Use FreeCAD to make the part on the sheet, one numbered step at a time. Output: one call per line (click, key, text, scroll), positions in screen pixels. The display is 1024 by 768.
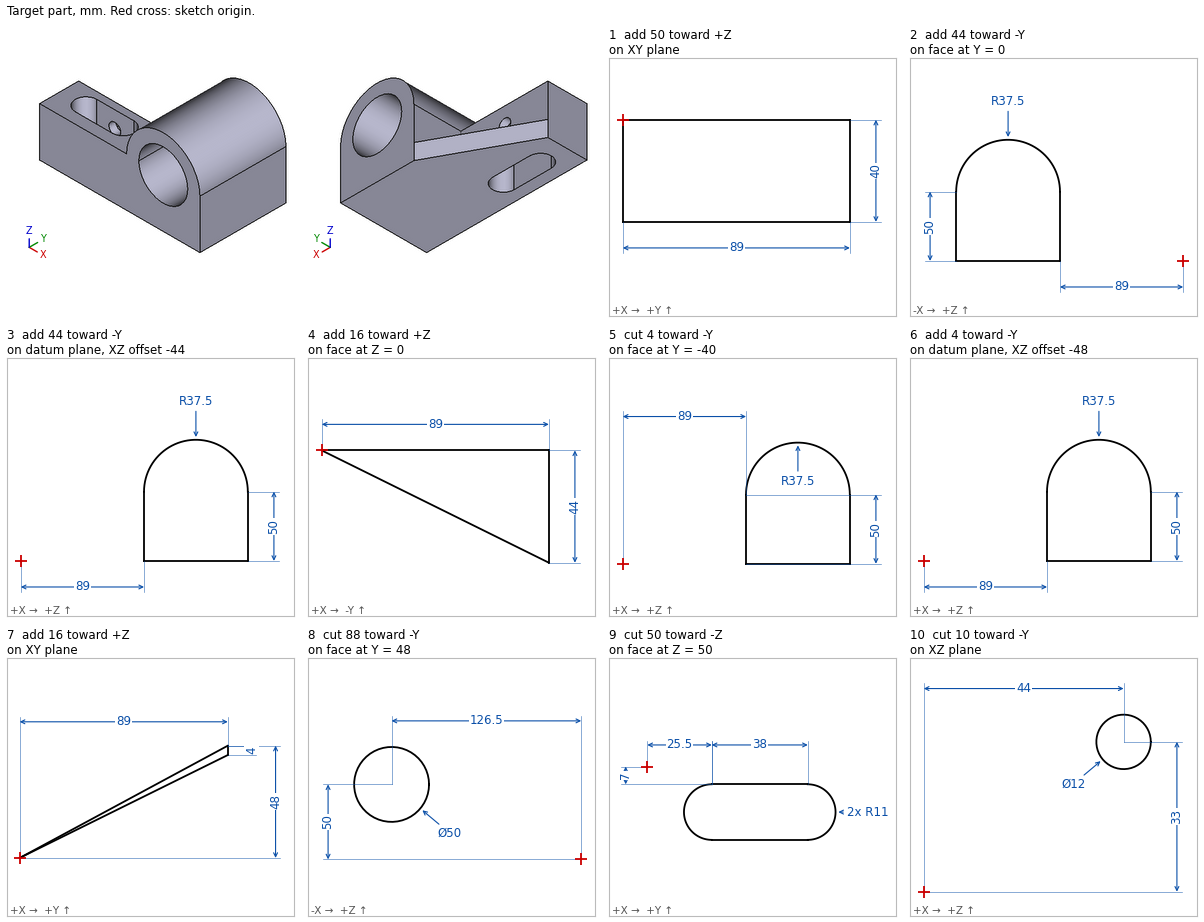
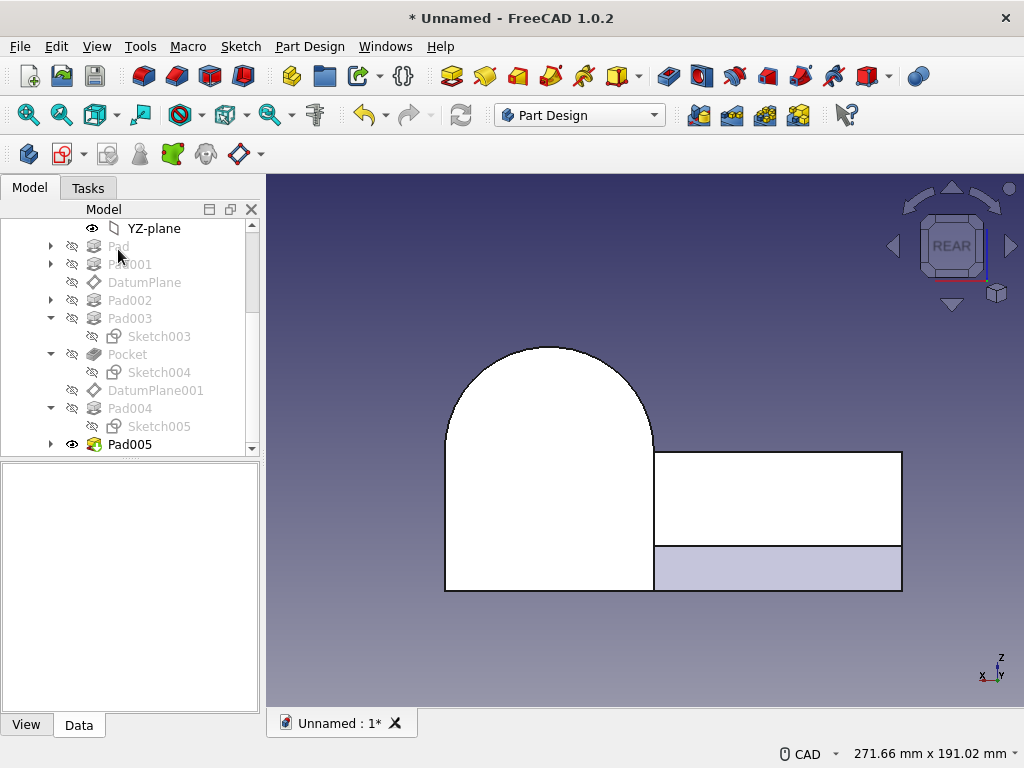
click(549, 468)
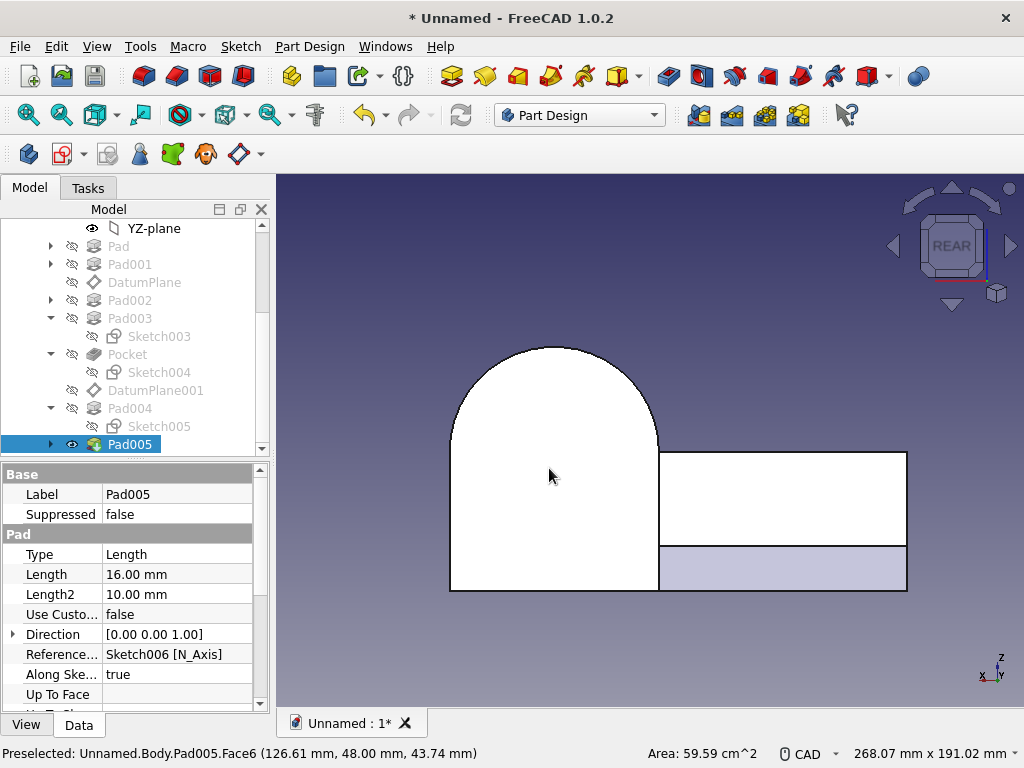
click(62, 154)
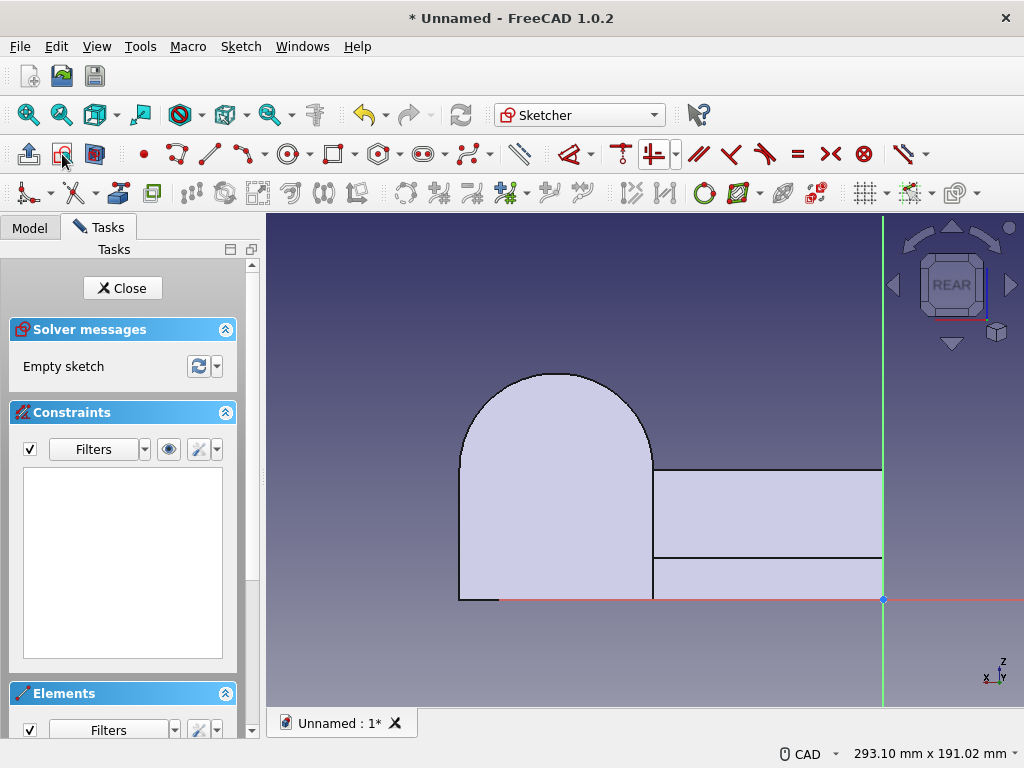
scroll(540, 479, up, 4)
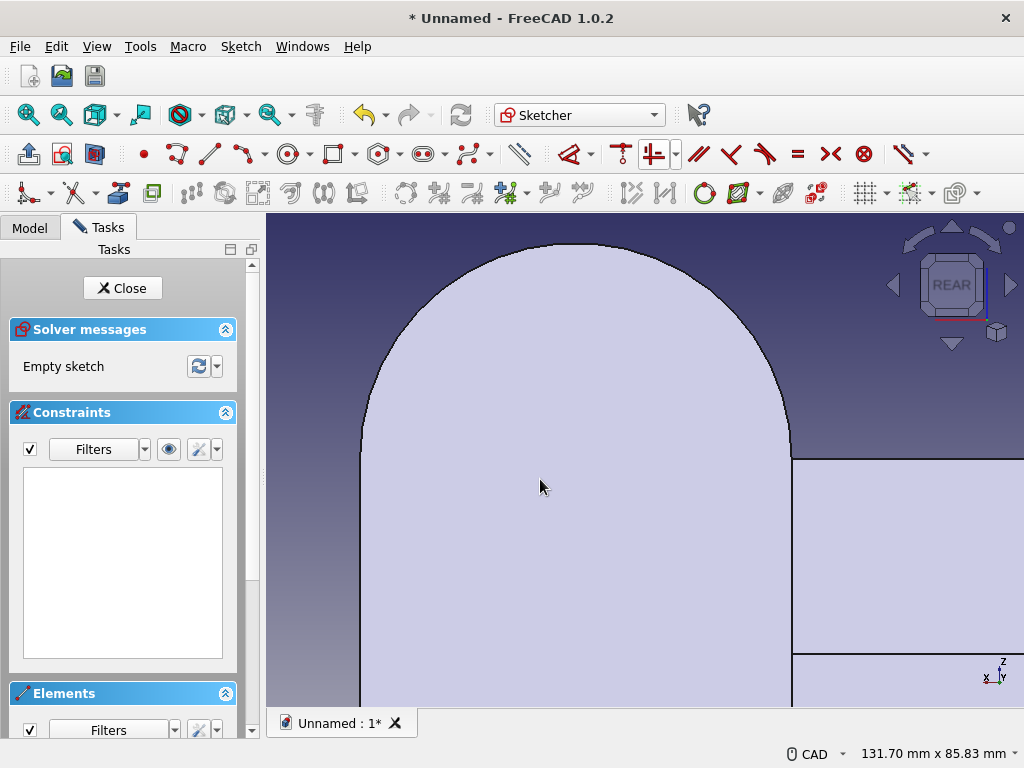
click(288, 154)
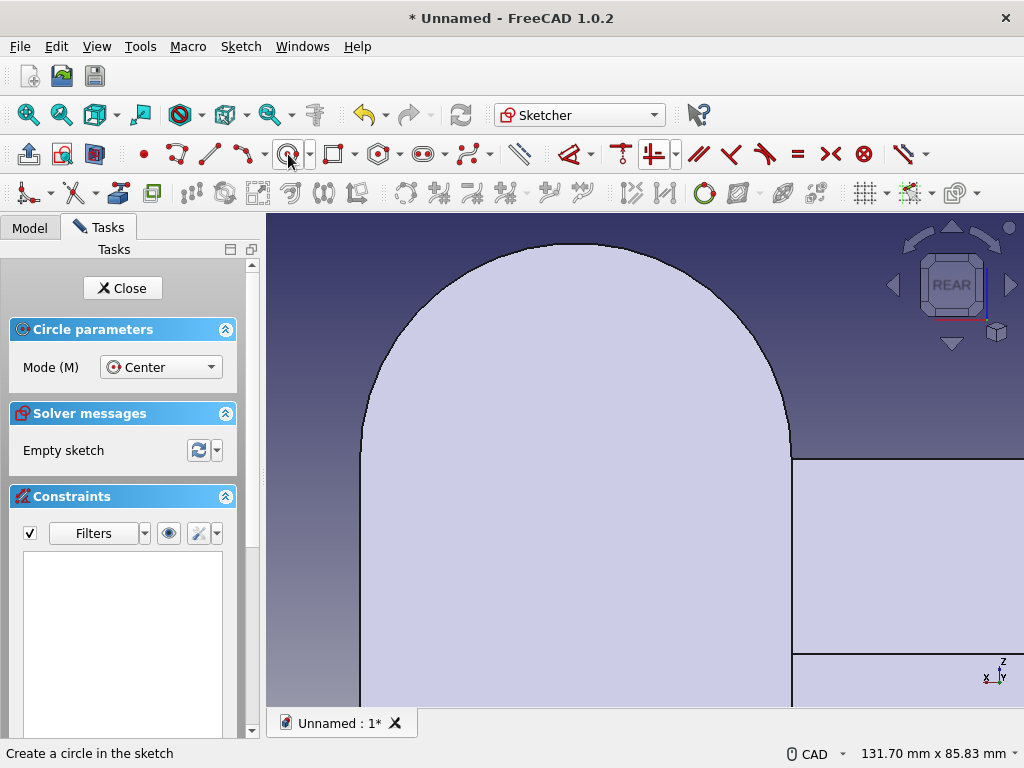
click(576, 459)
move(678, 357)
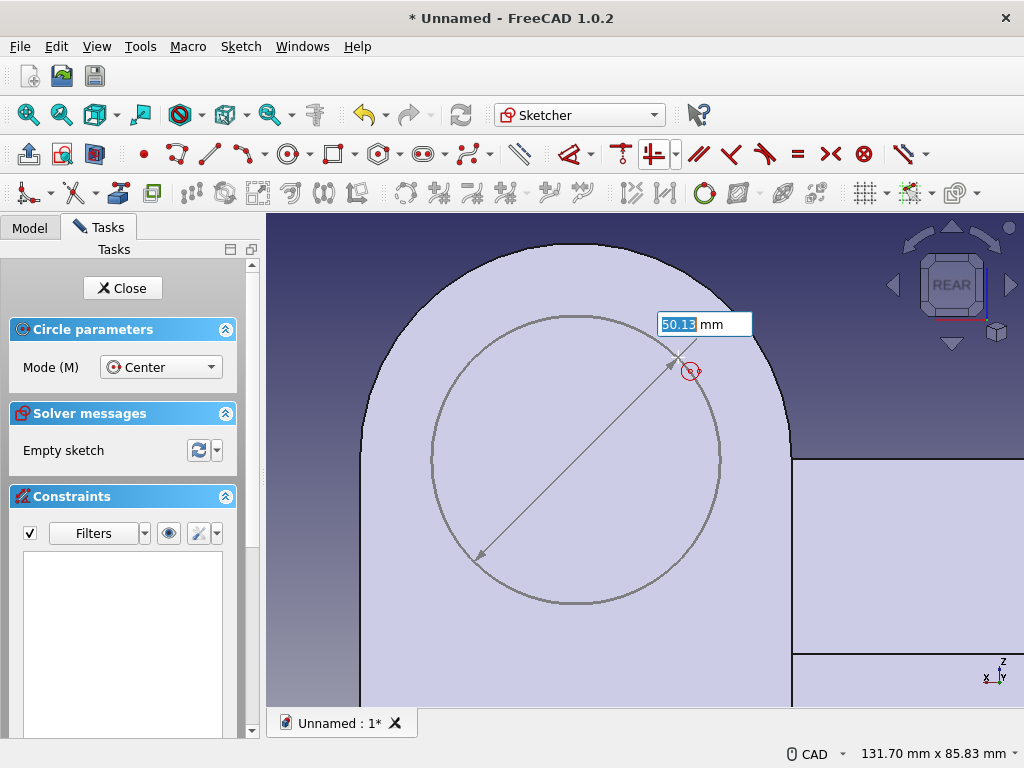
text(50)
key(Return)
key(Escape)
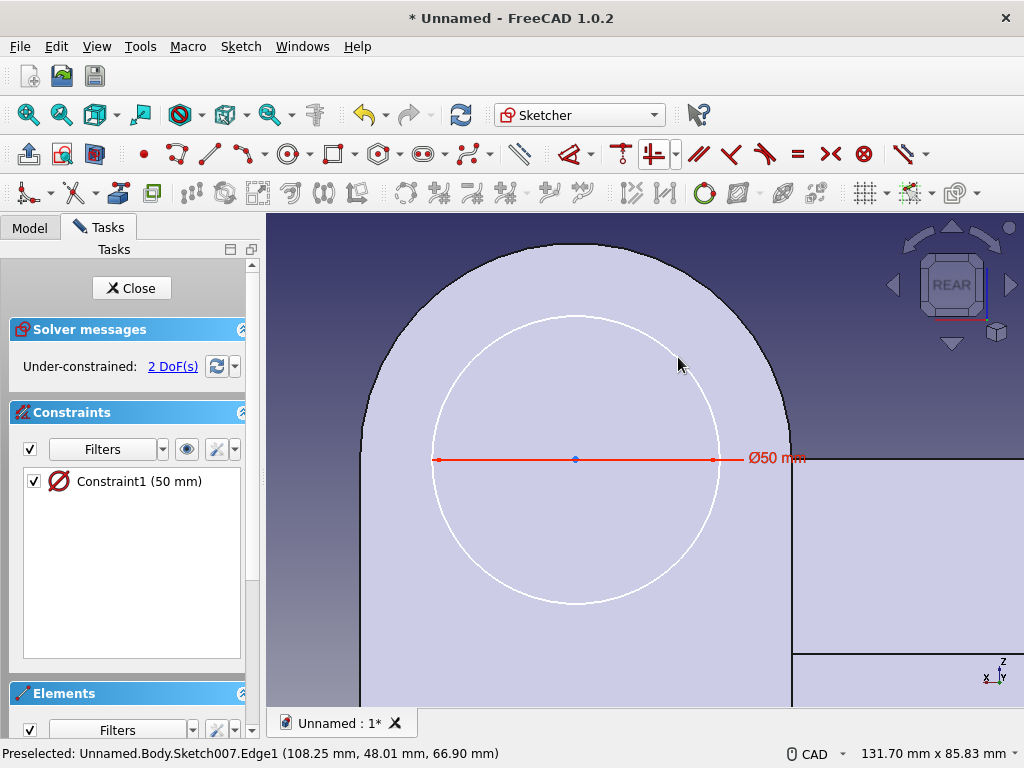
click(568, 154)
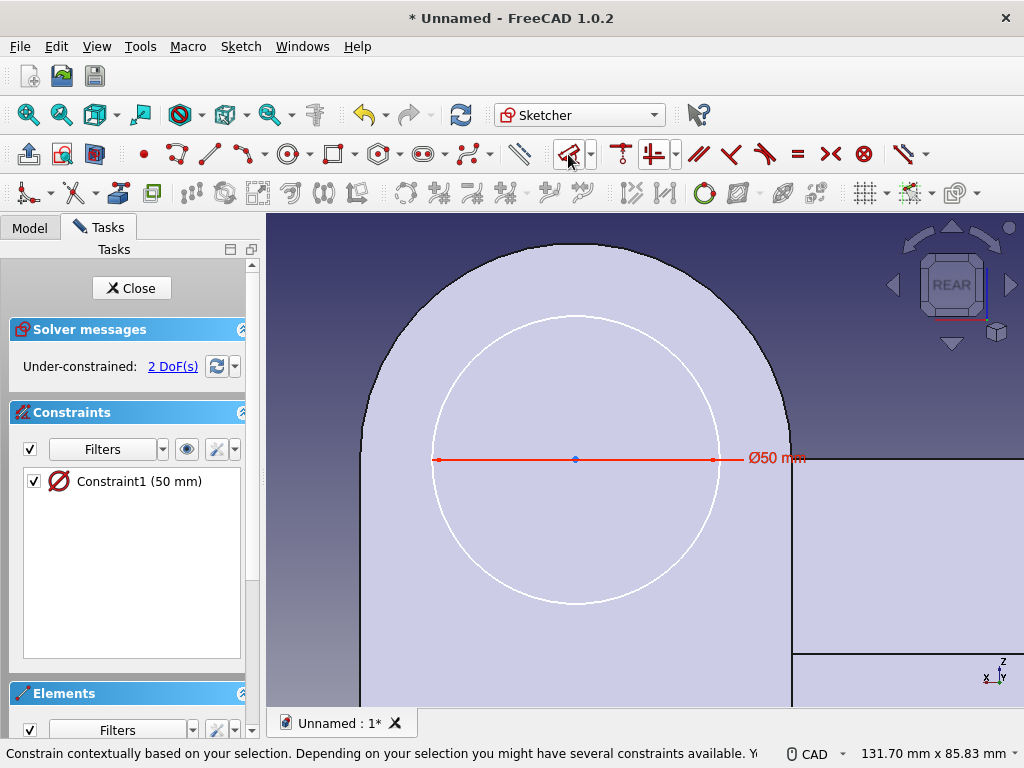
click(576, 460)
click(542, 570)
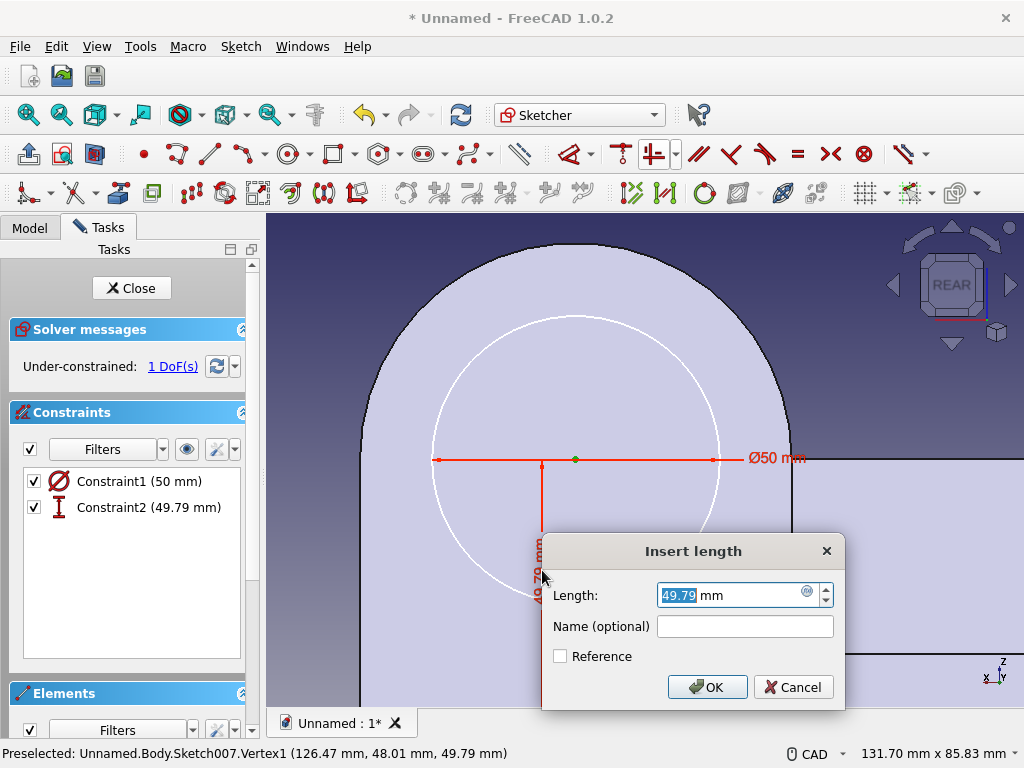
text(50)
key(Return)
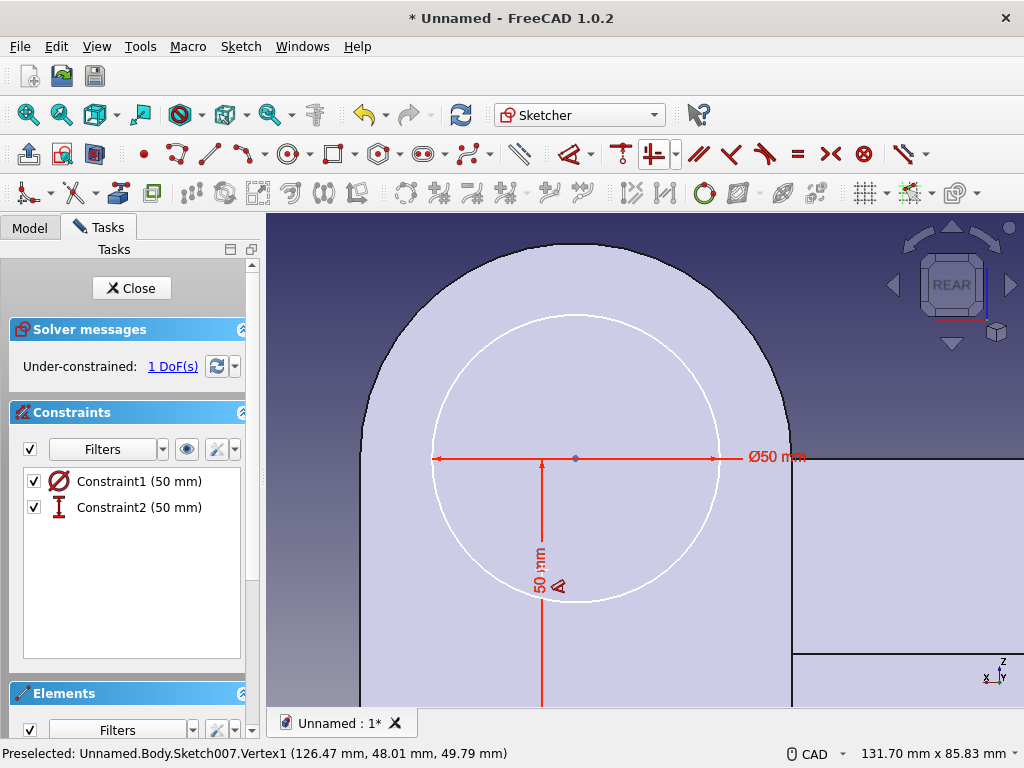
click(576, 459)
click(652, 425)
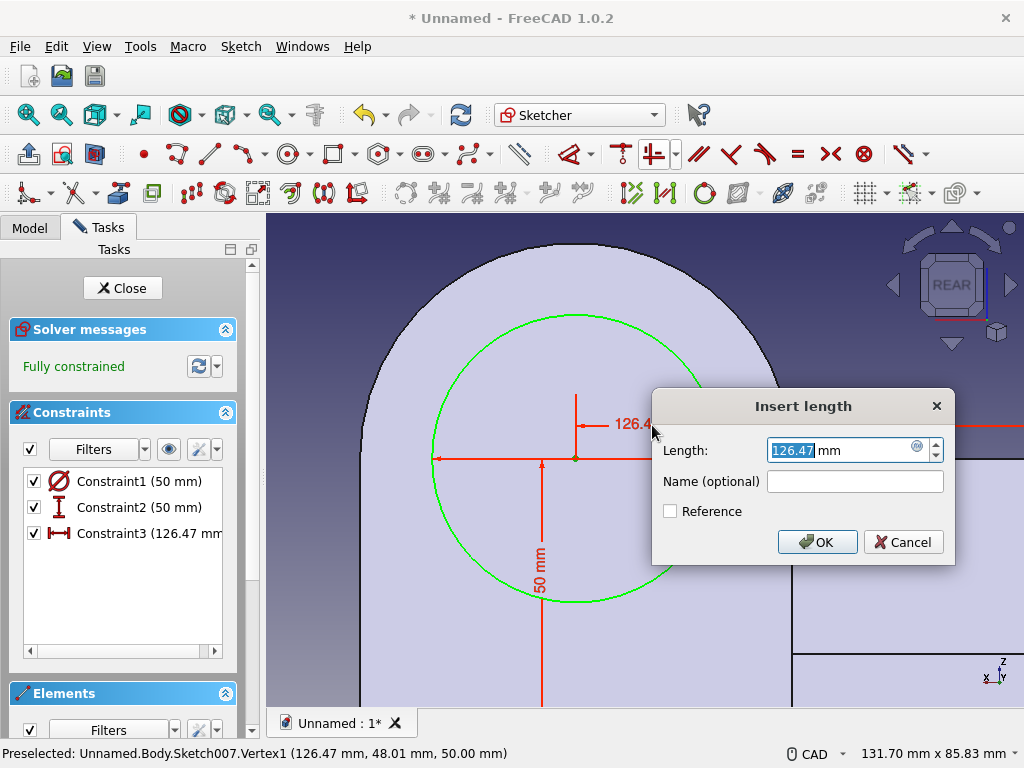
text(126.5)
key(Return)
key(Escape)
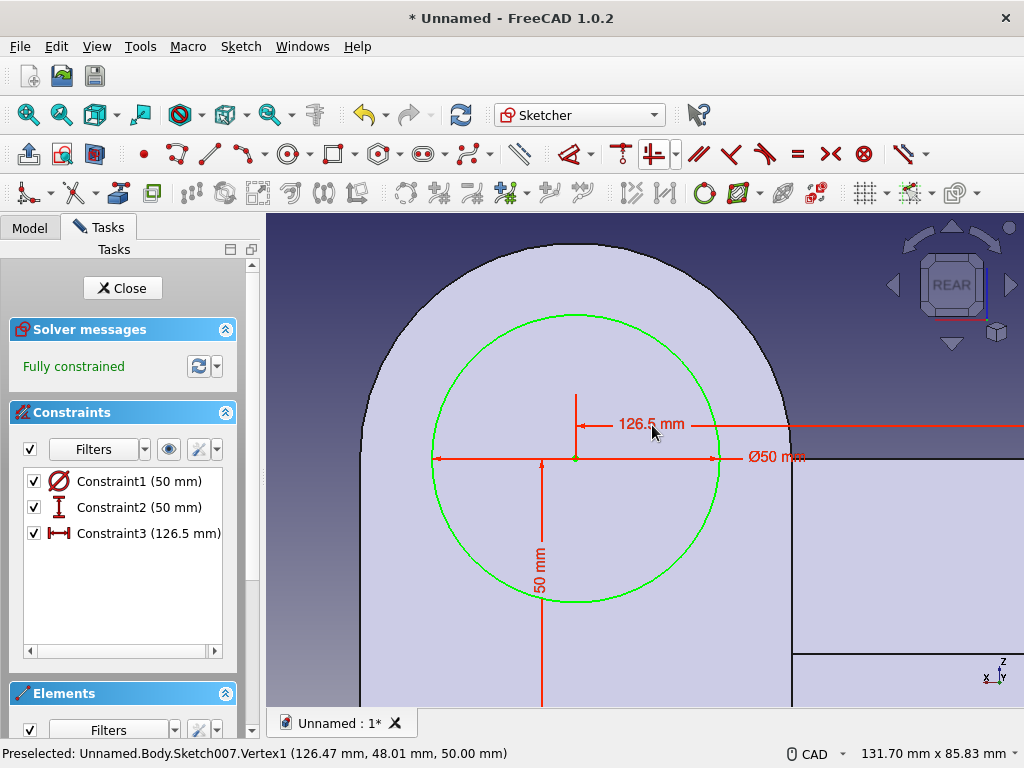
click(123, 288)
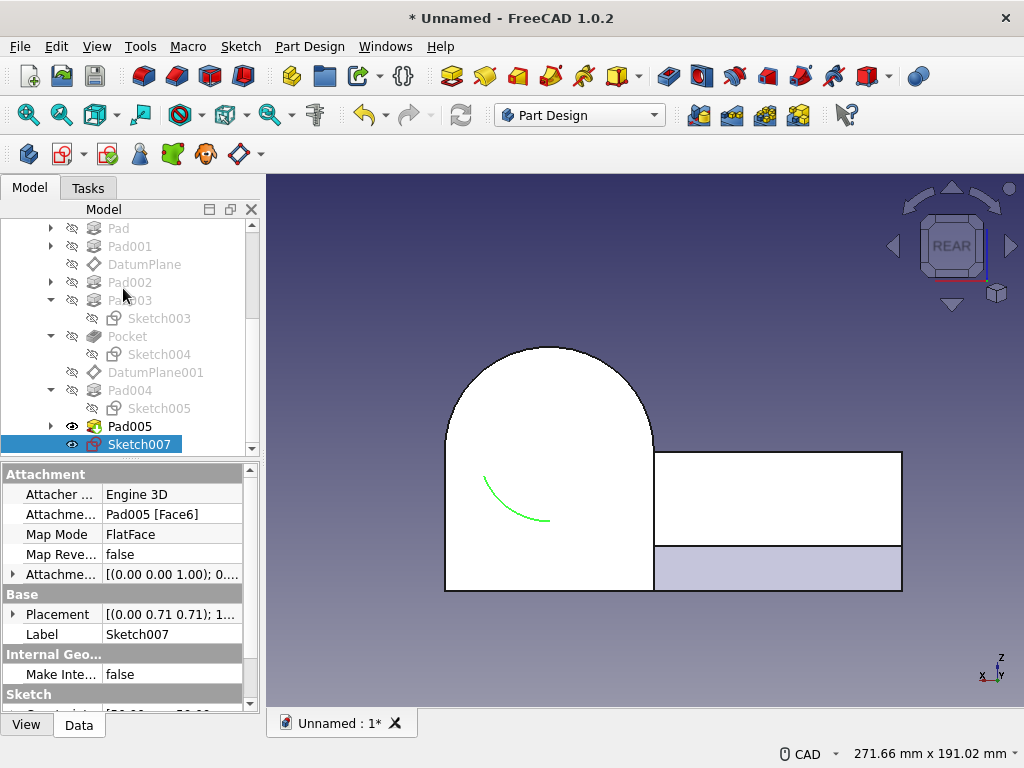
click(669, 76)